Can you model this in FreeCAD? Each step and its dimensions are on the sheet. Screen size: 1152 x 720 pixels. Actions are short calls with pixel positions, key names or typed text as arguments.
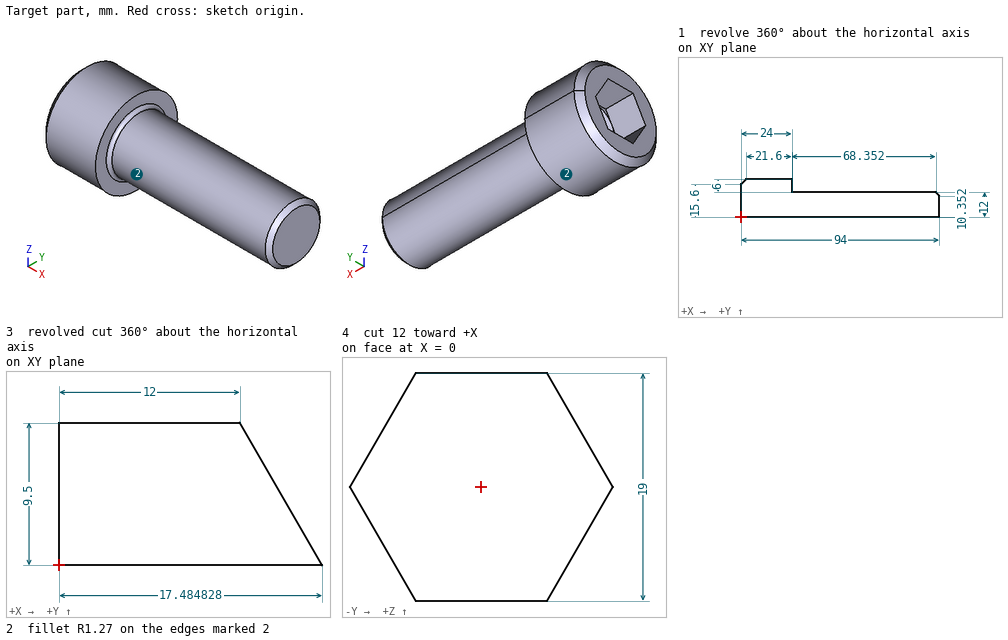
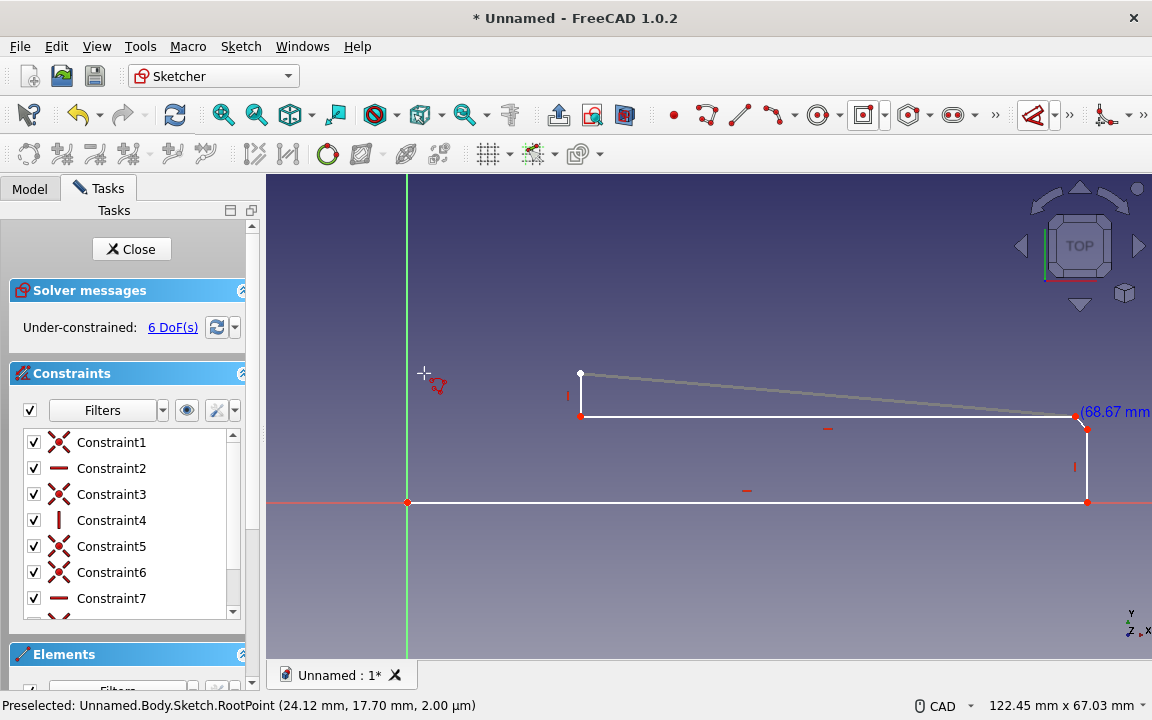
click(425, 373)
click(416, 390)
click(407, 503)
key(Escape)
key(Escape)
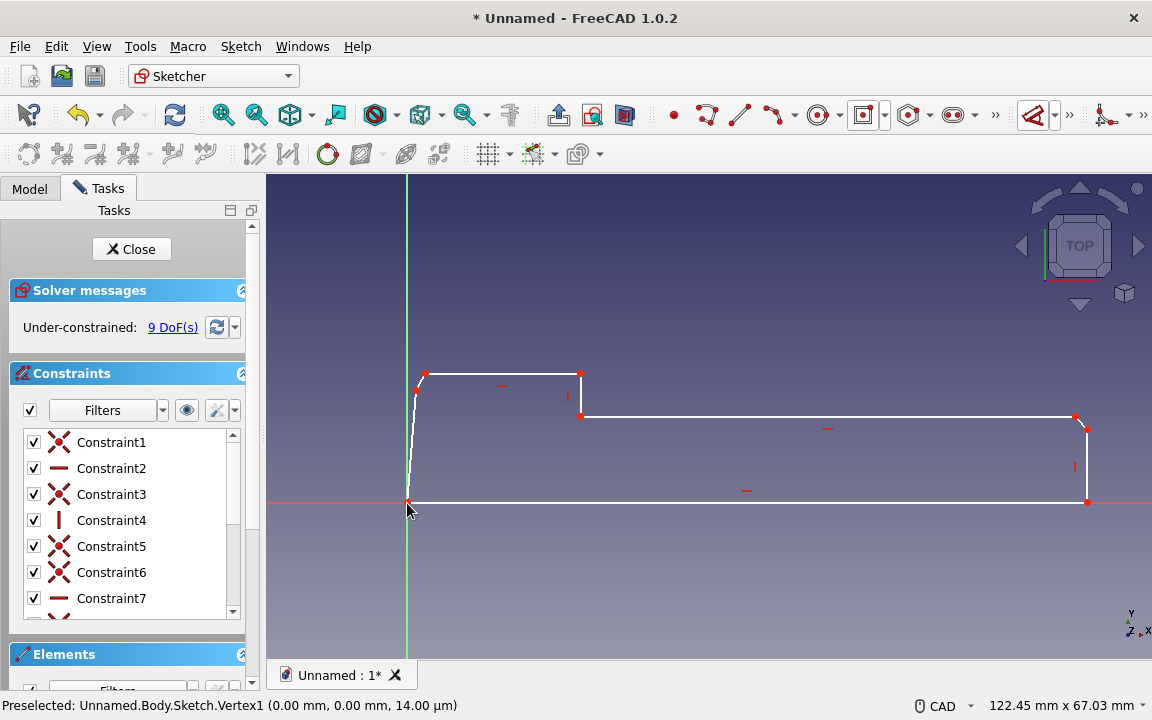
click(410, 469)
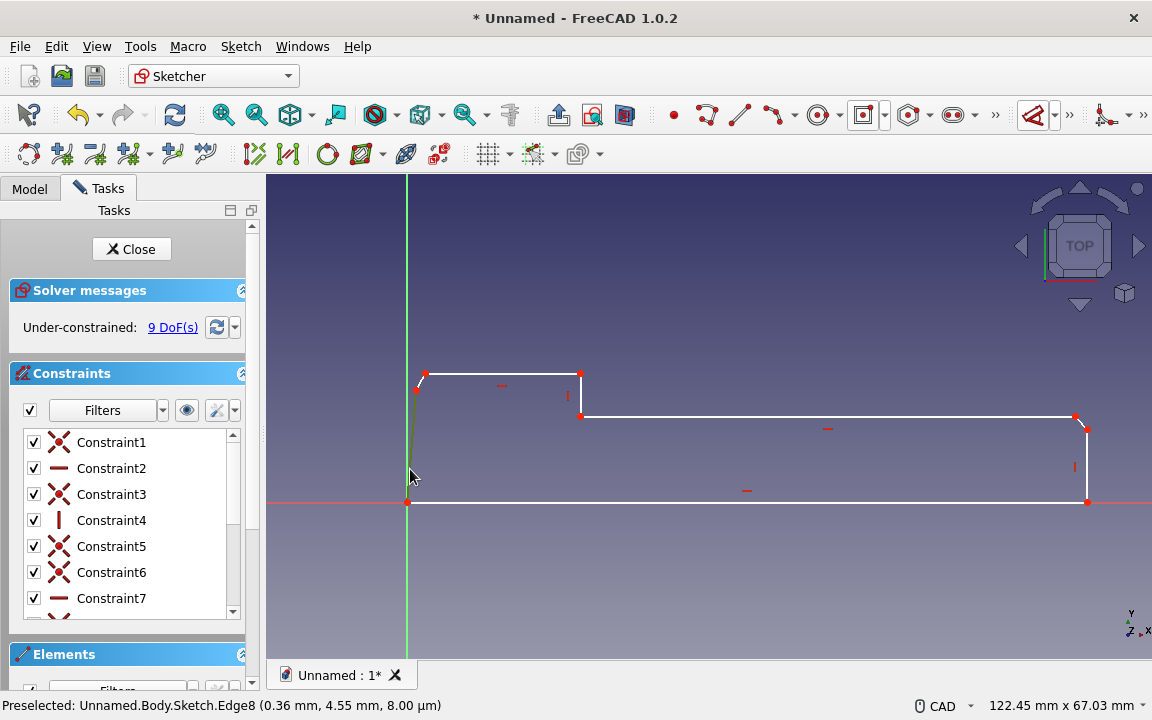
key(v)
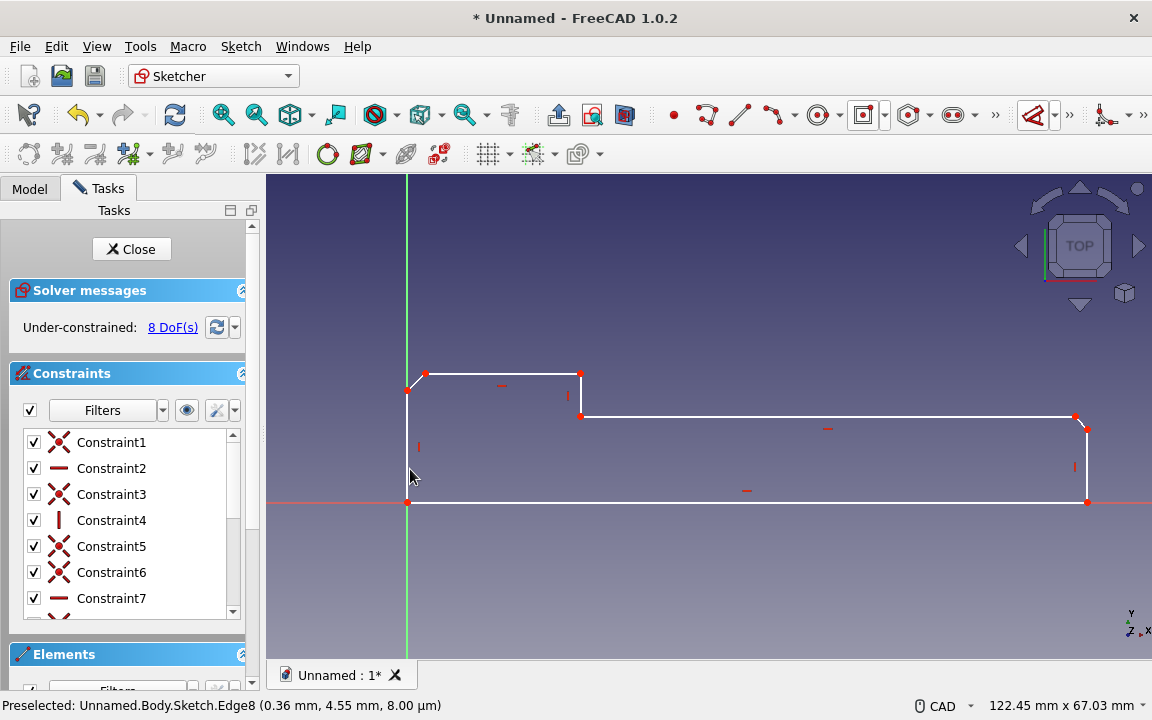
click(581, 404)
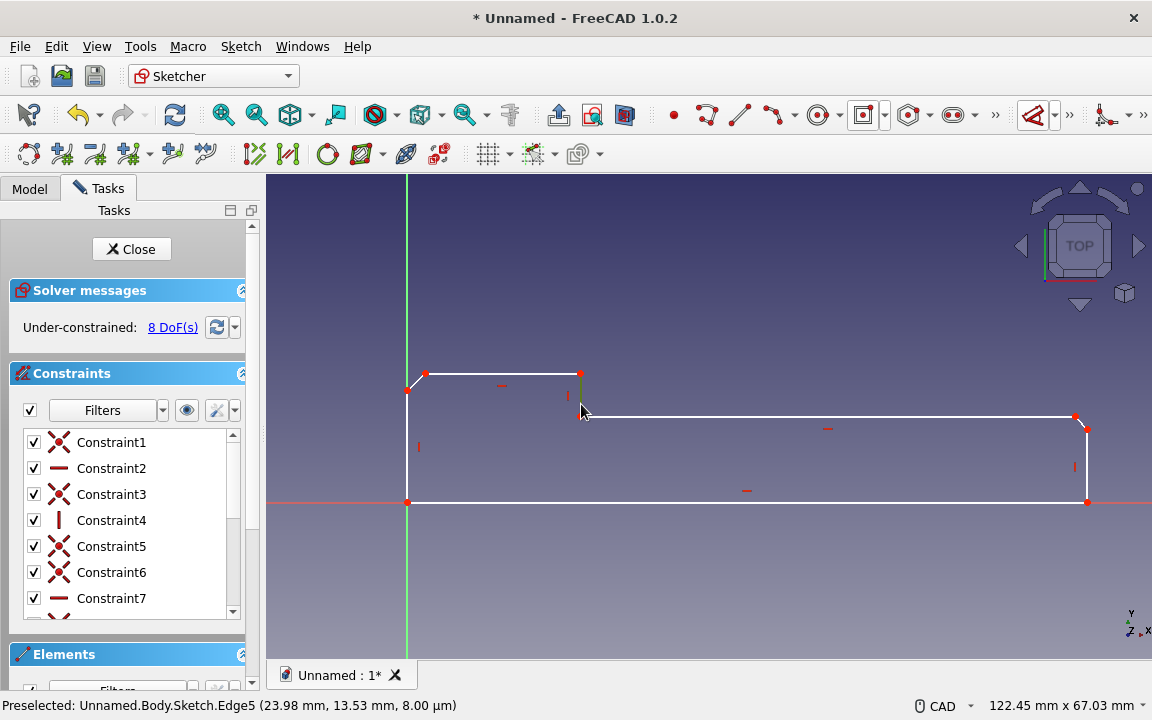
click(1054, 116)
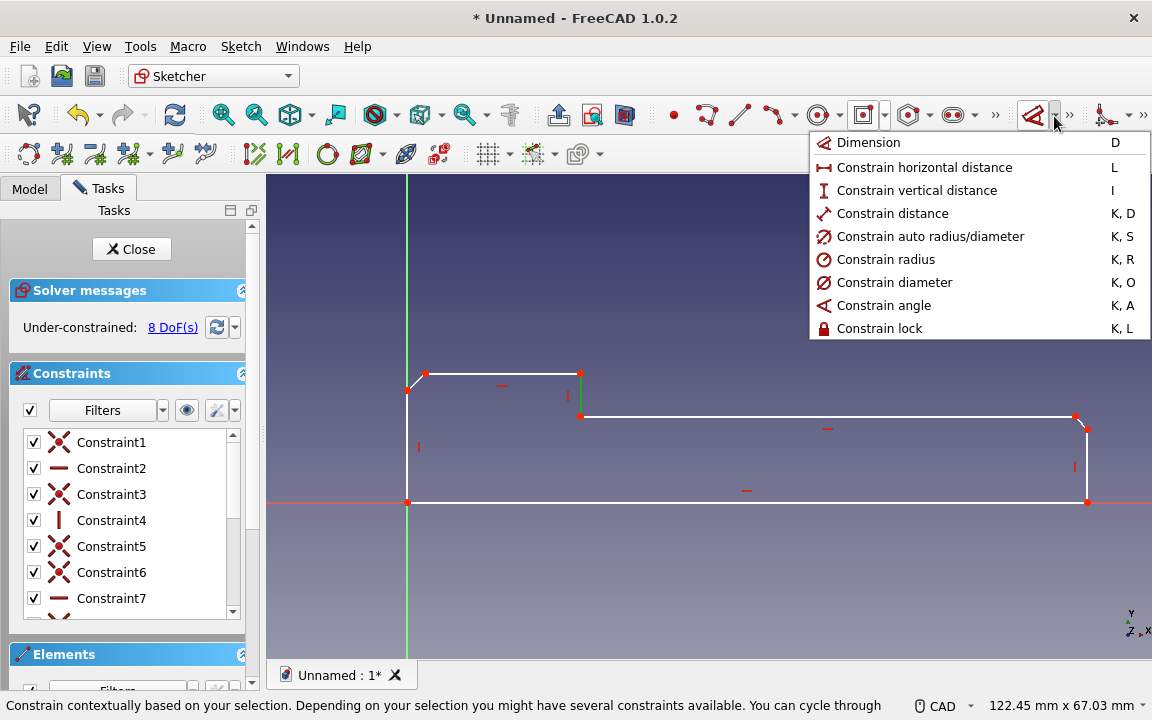
click(980, 190)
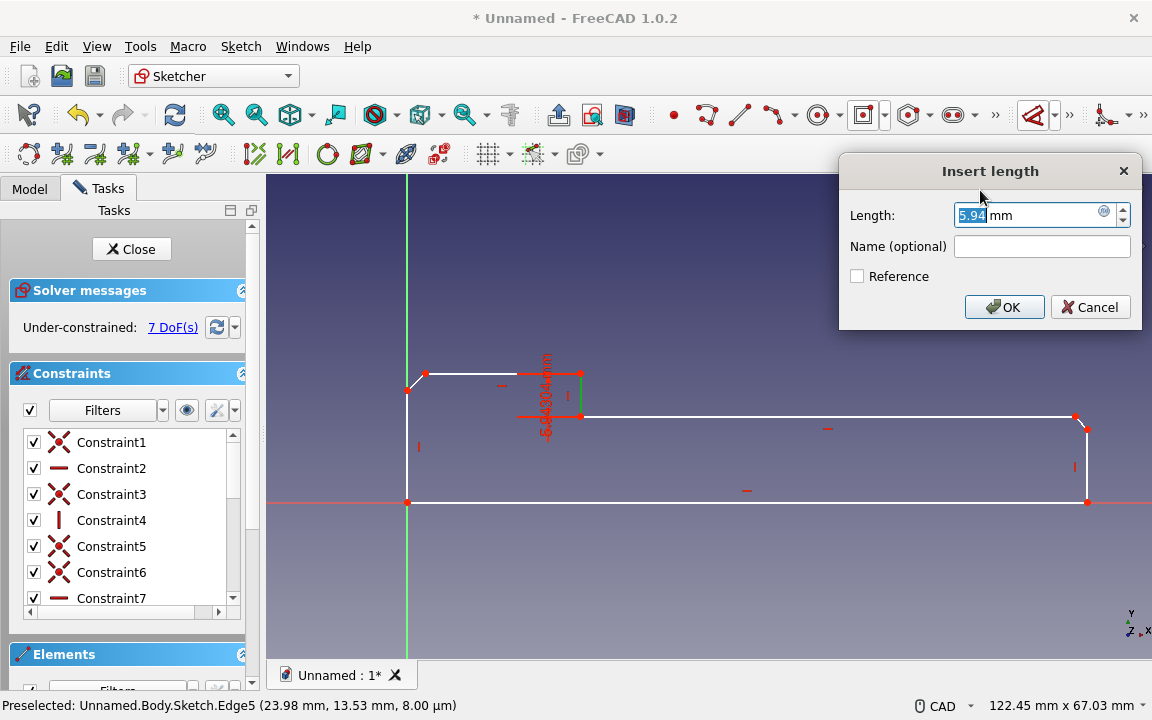
text(6)
key(Return)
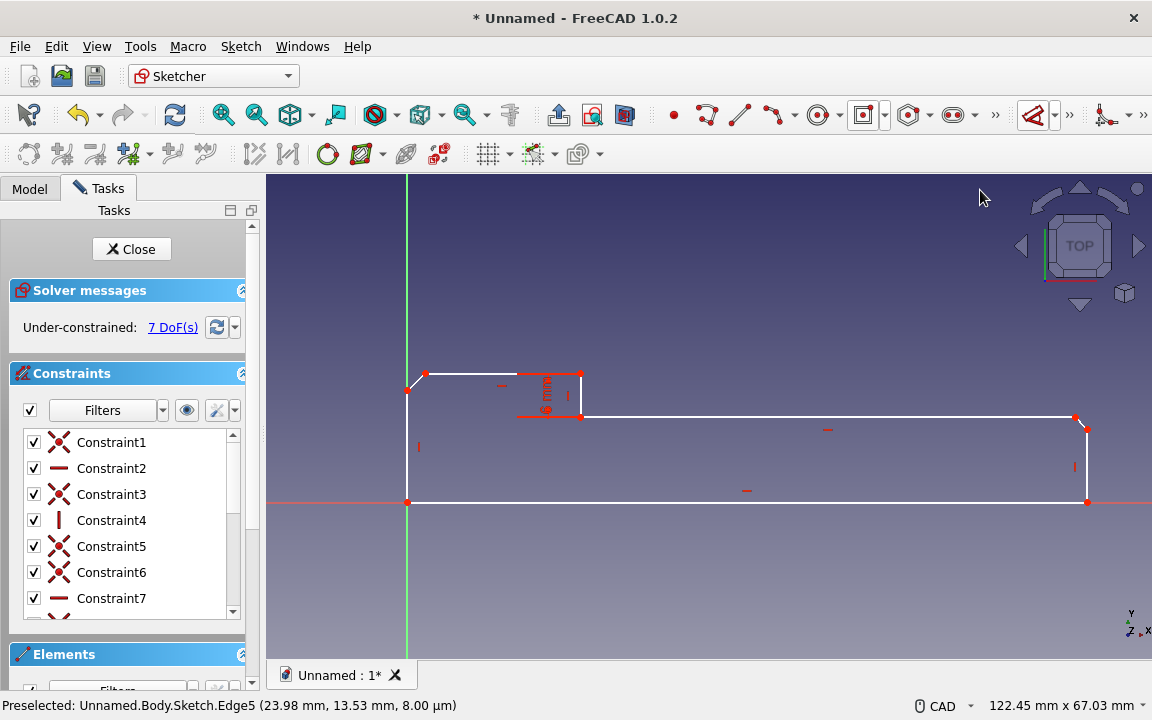
click(611, 503)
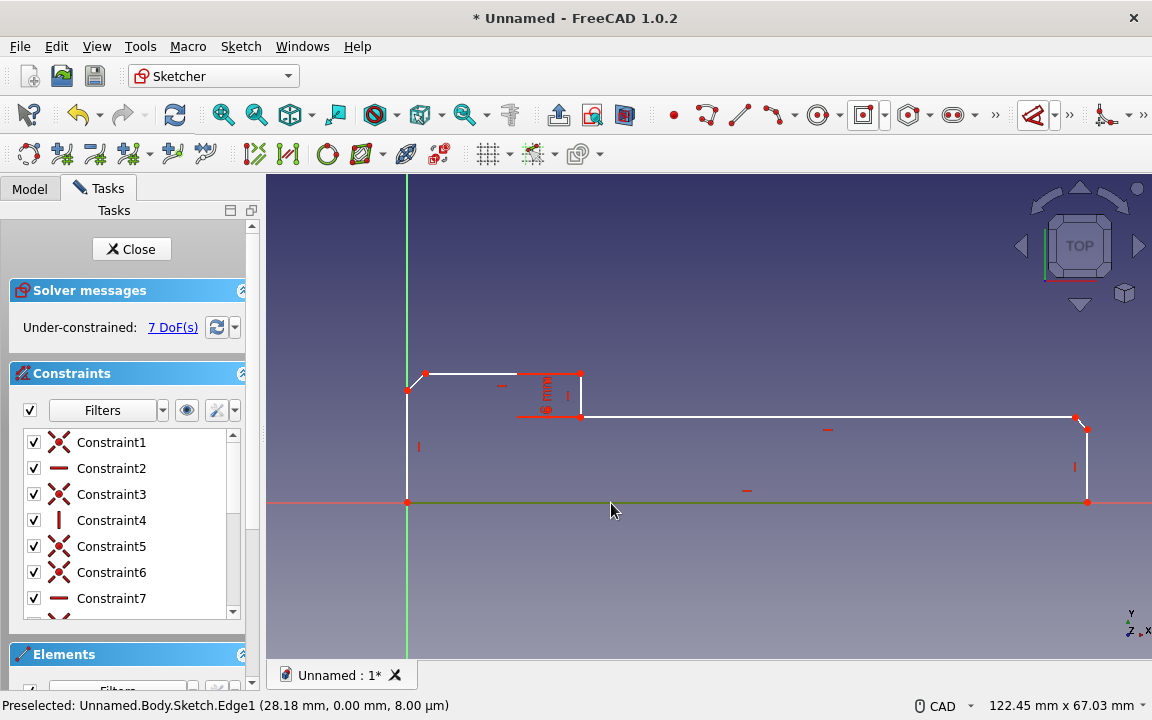
key(l)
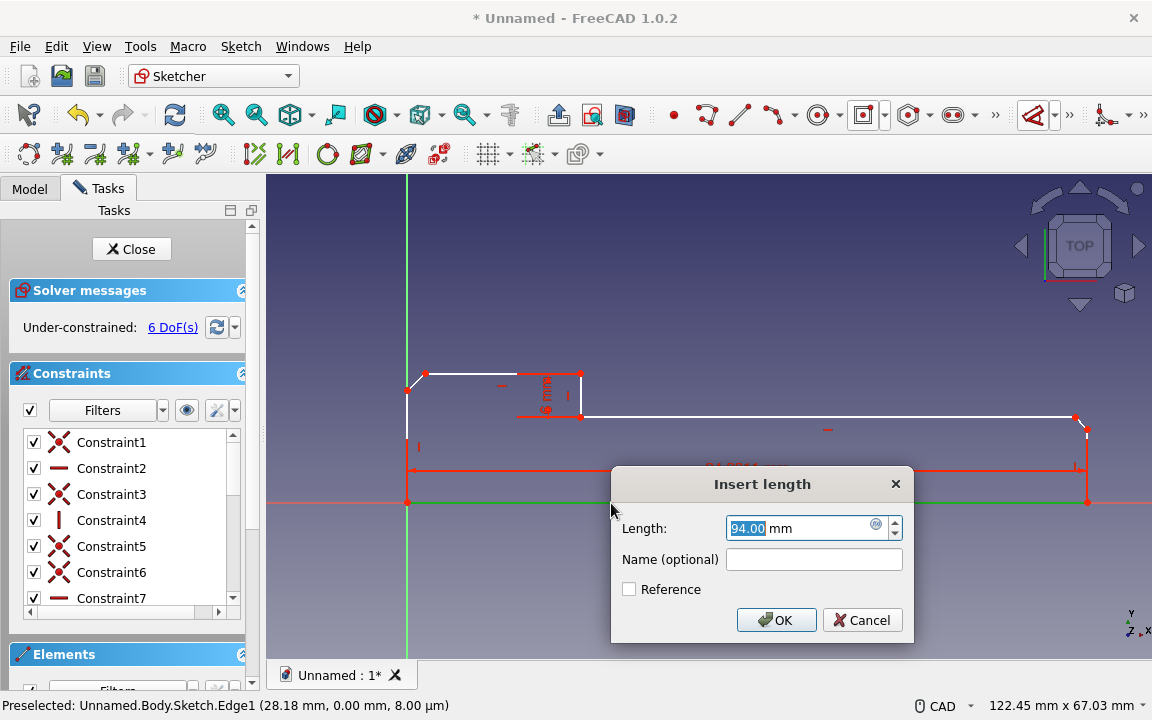
text(94)
key(Return)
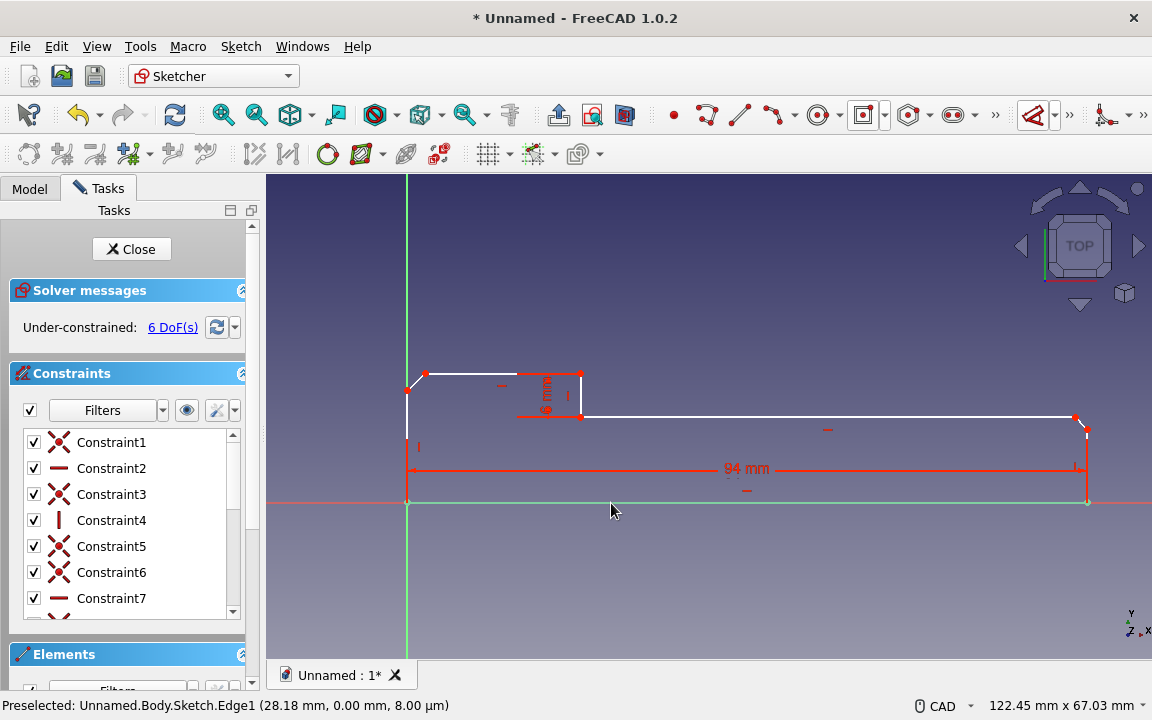
scroll(424, 373, down, 2)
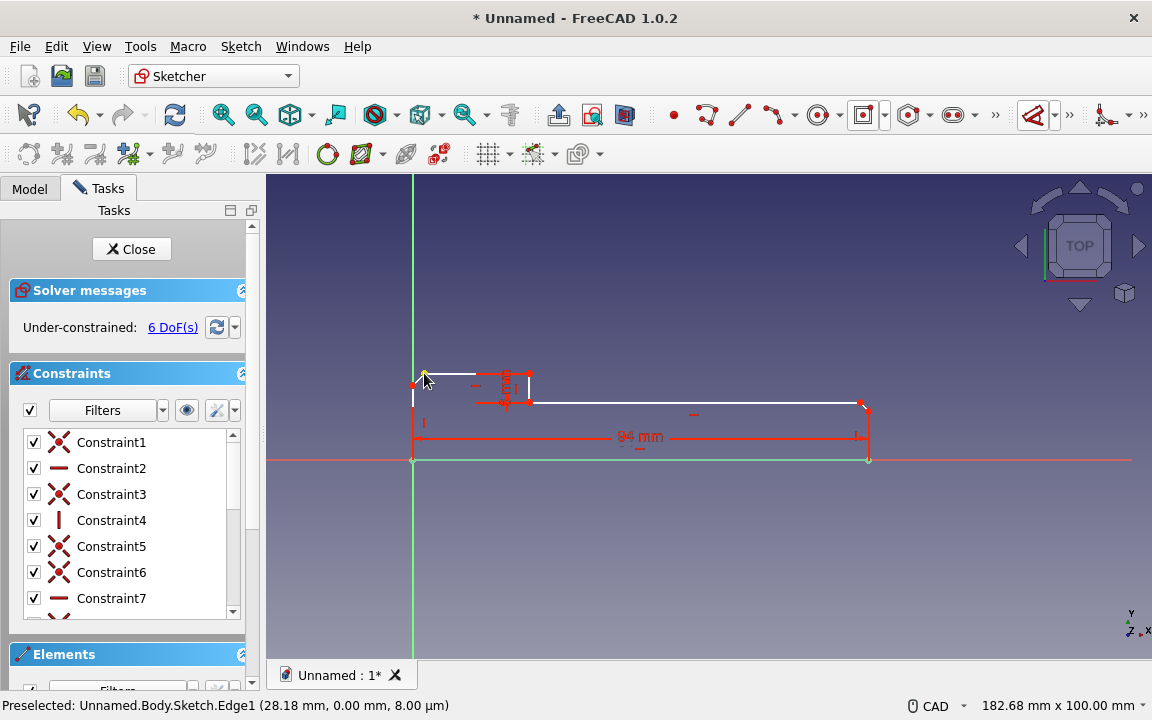
click(861, 403)